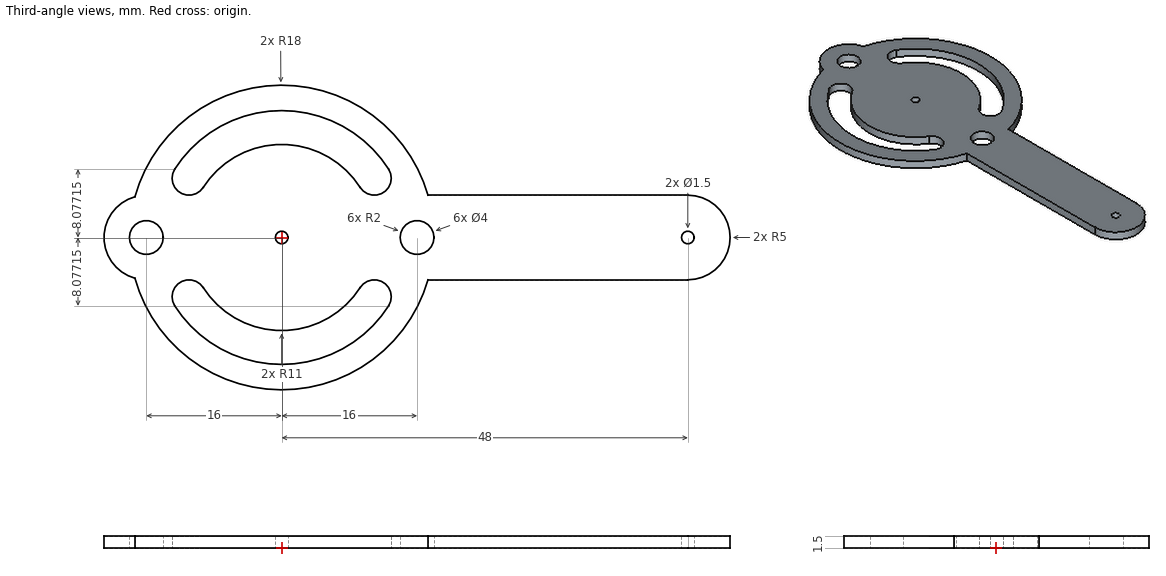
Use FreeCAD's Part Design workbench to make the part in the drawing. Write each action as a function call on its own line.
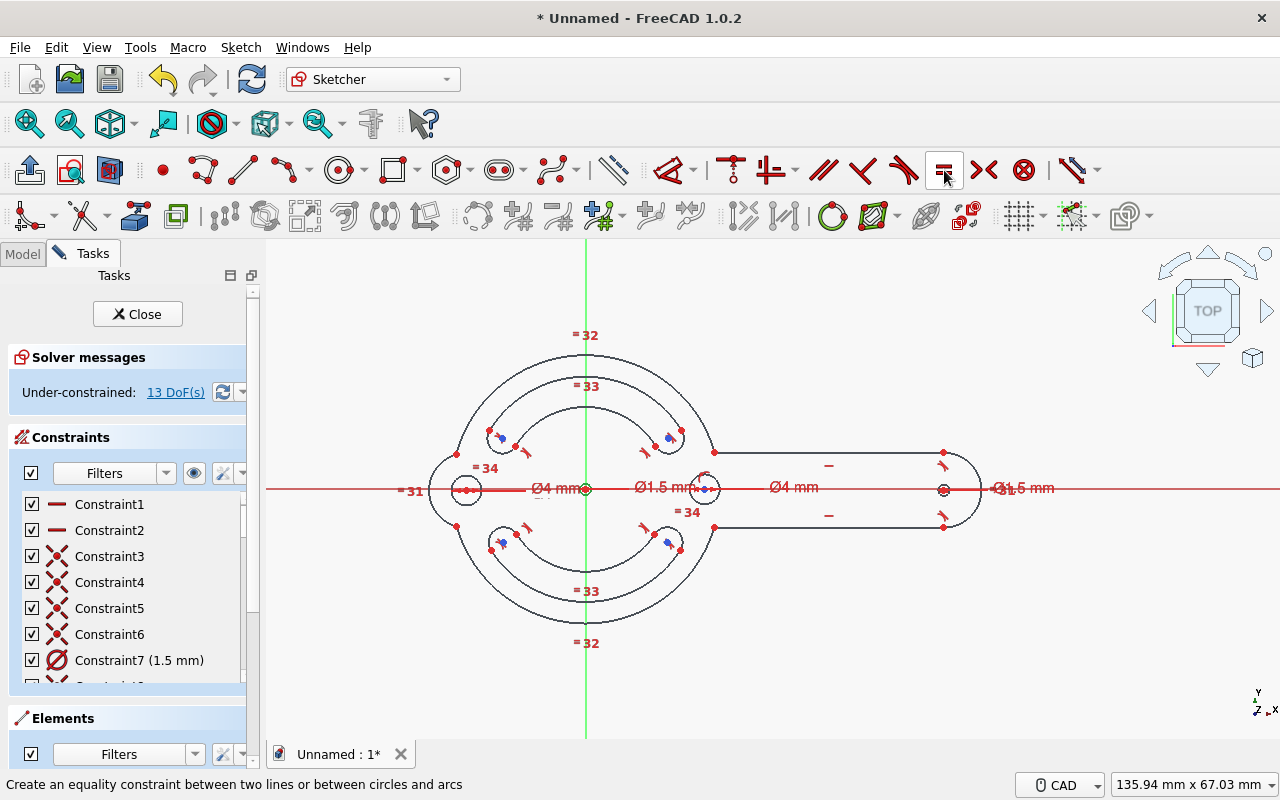
click(944, 490)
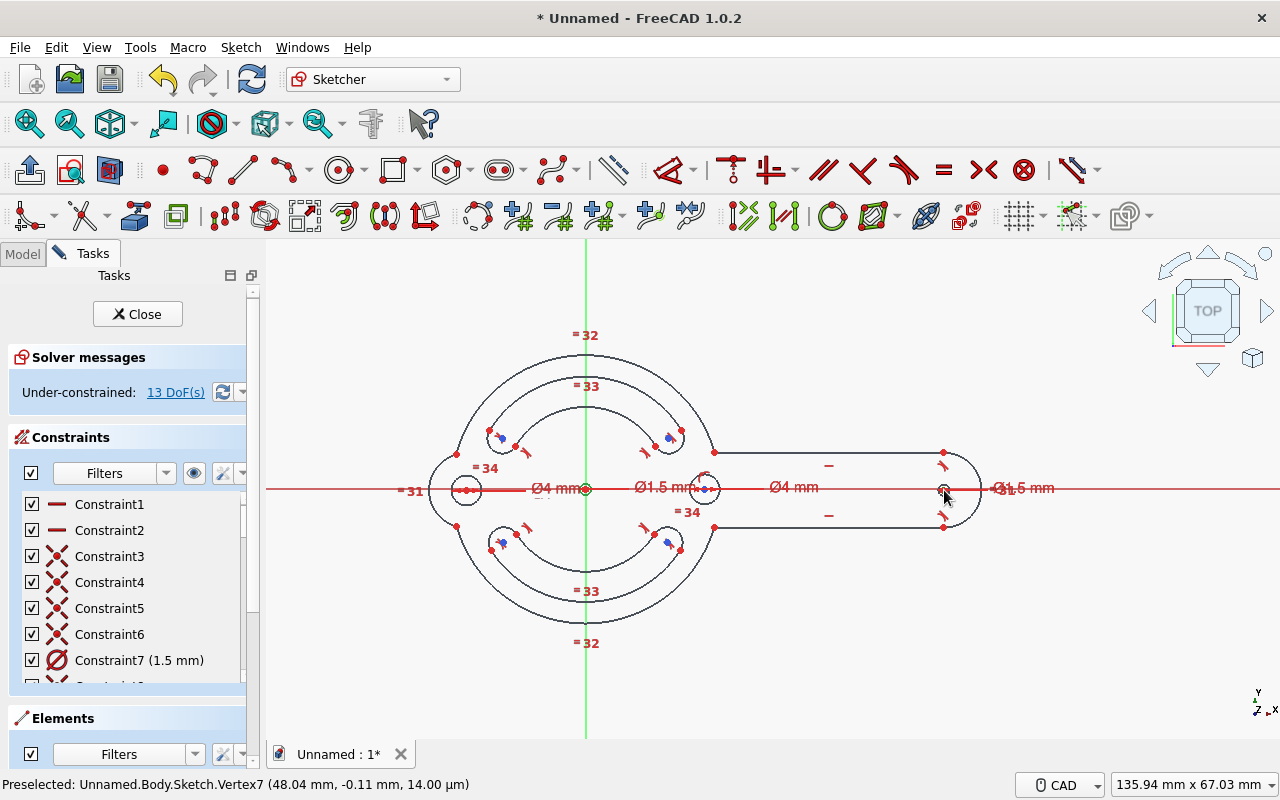
click(353, 489)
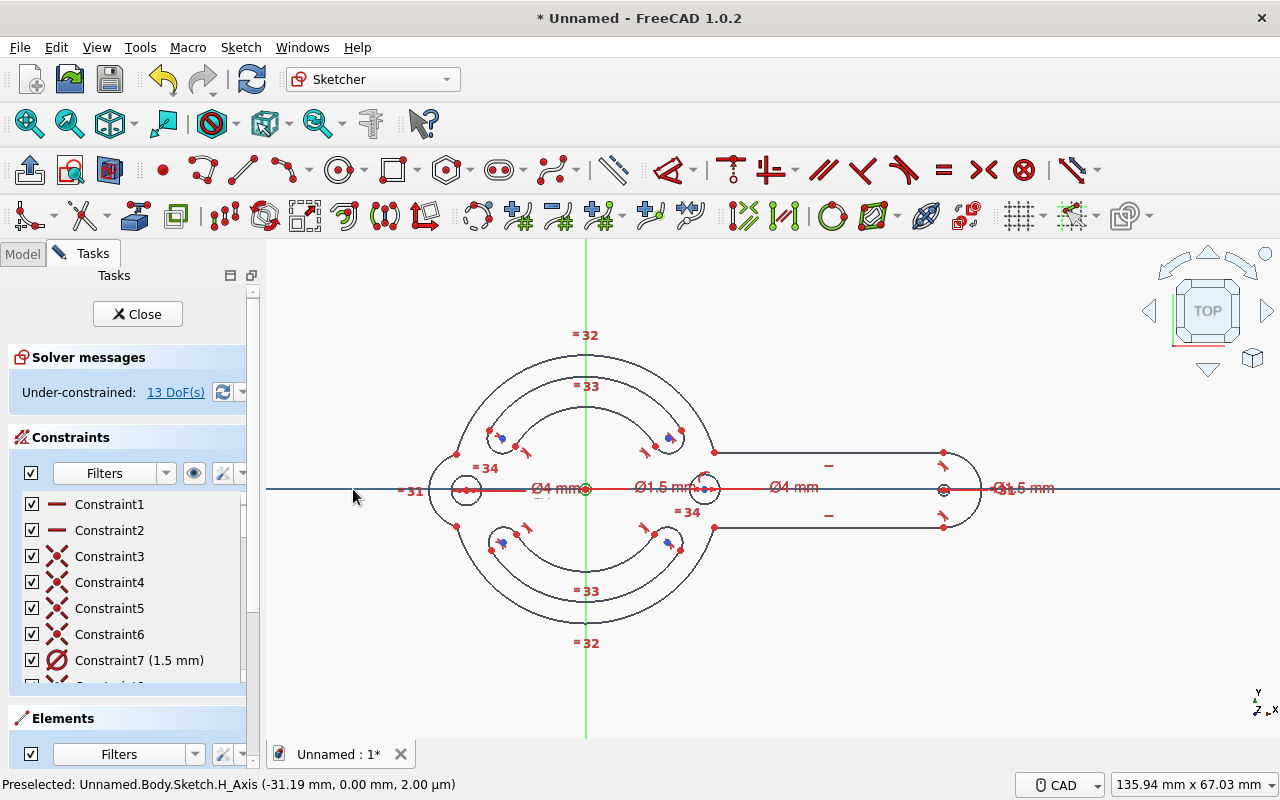
click(732, 170)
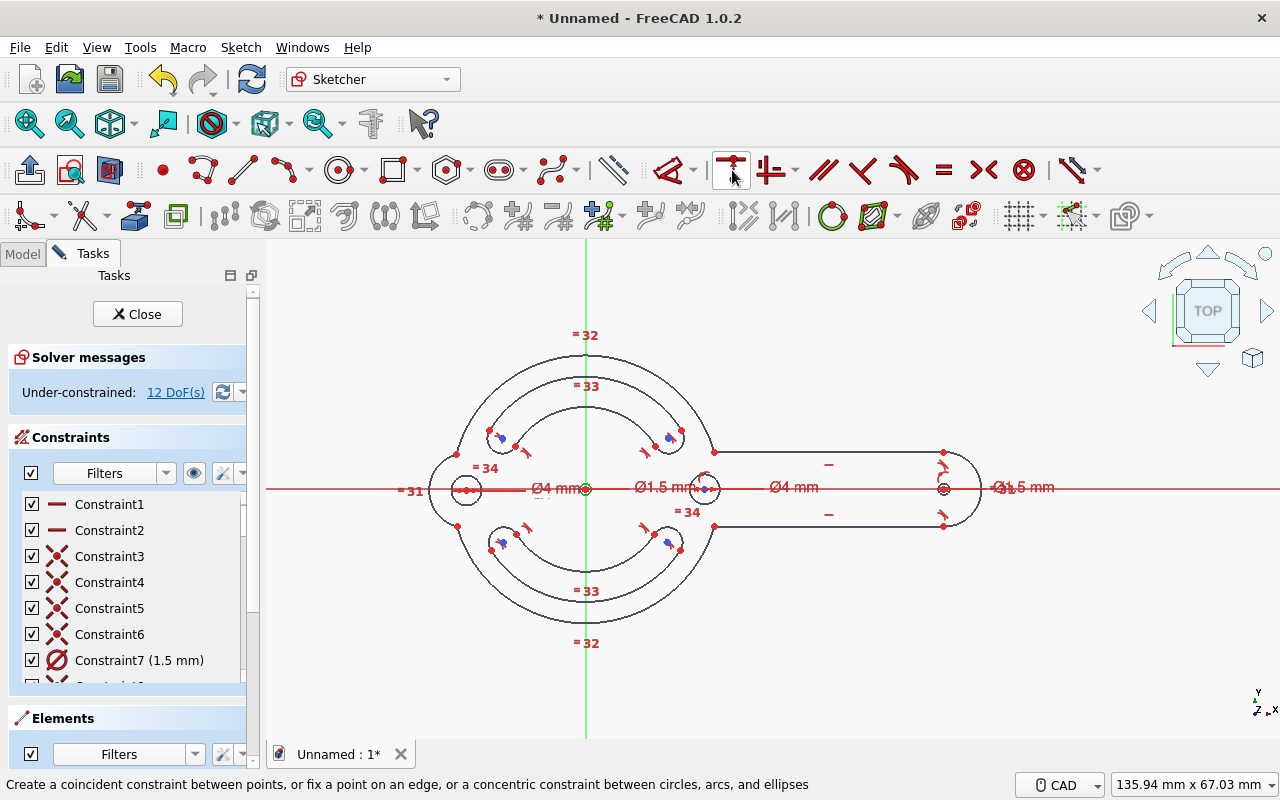
click(467, 491)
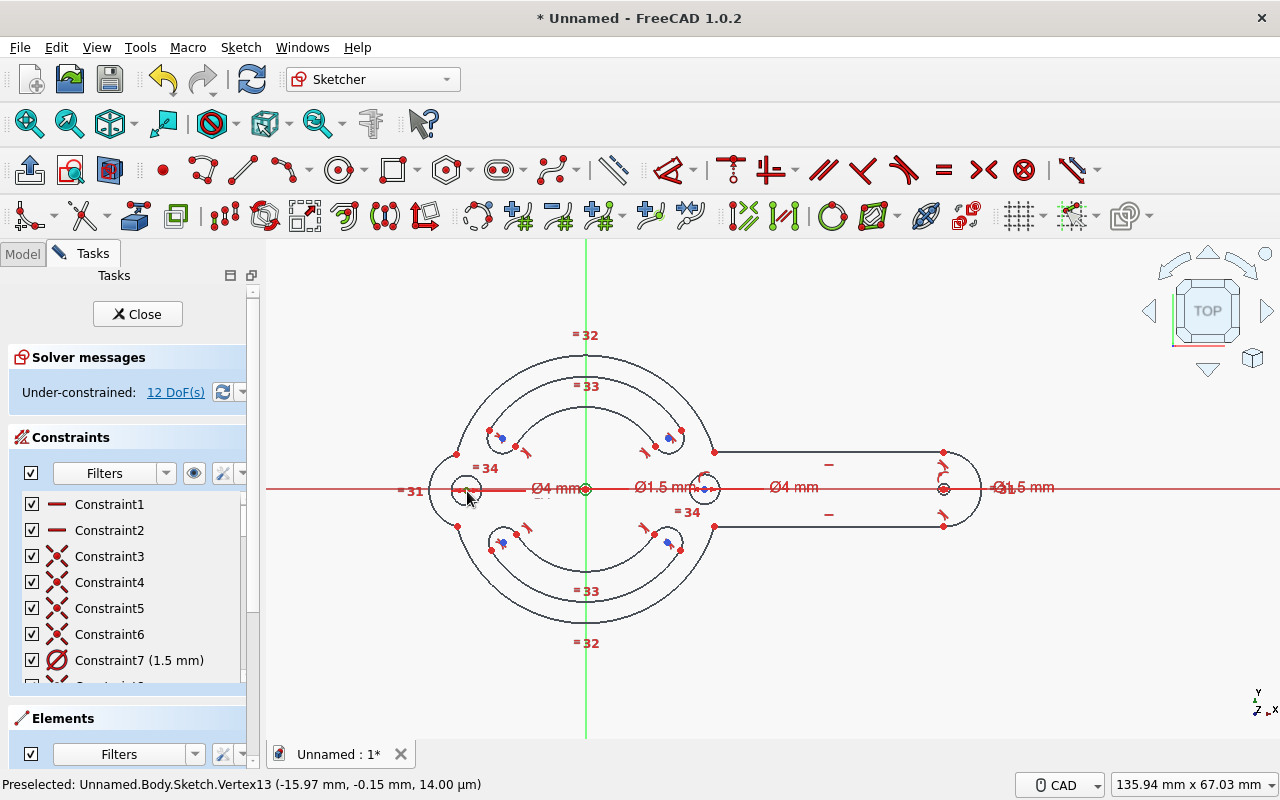
click(353, 489)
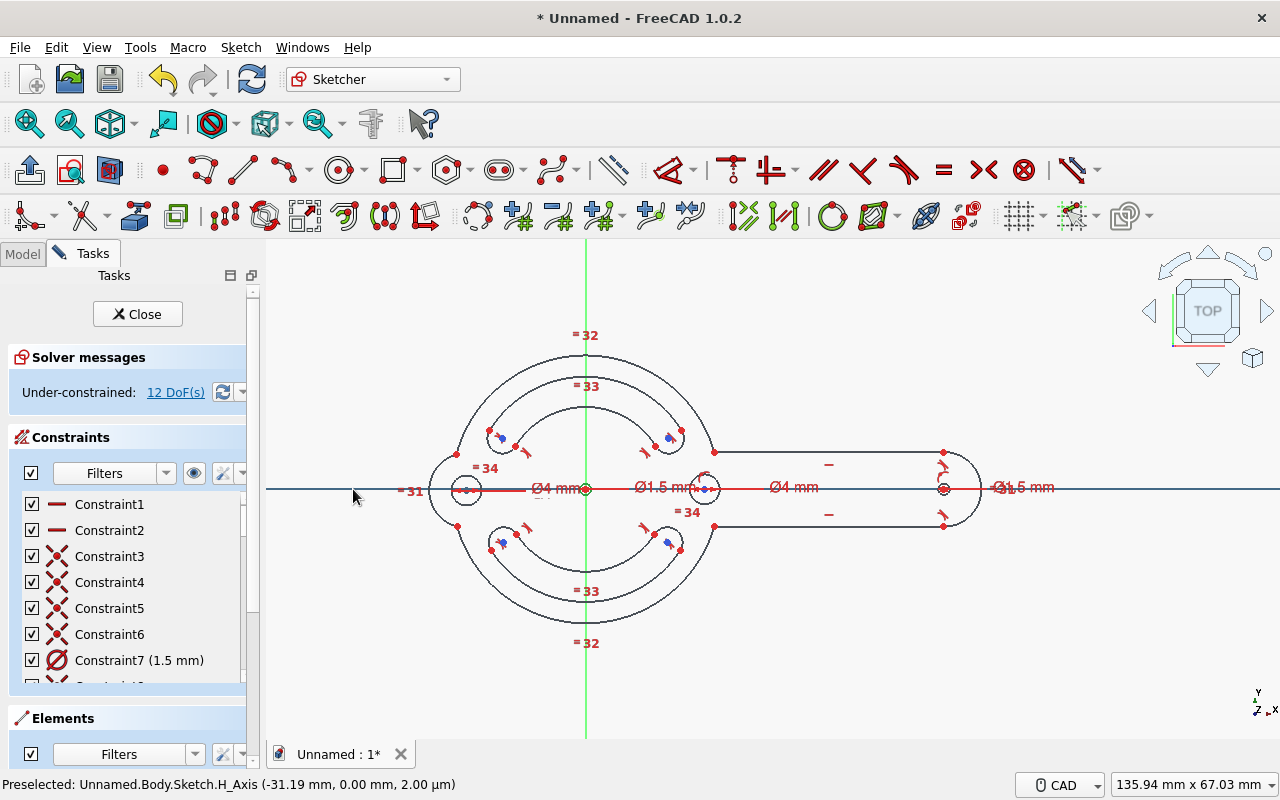
click(732, 170)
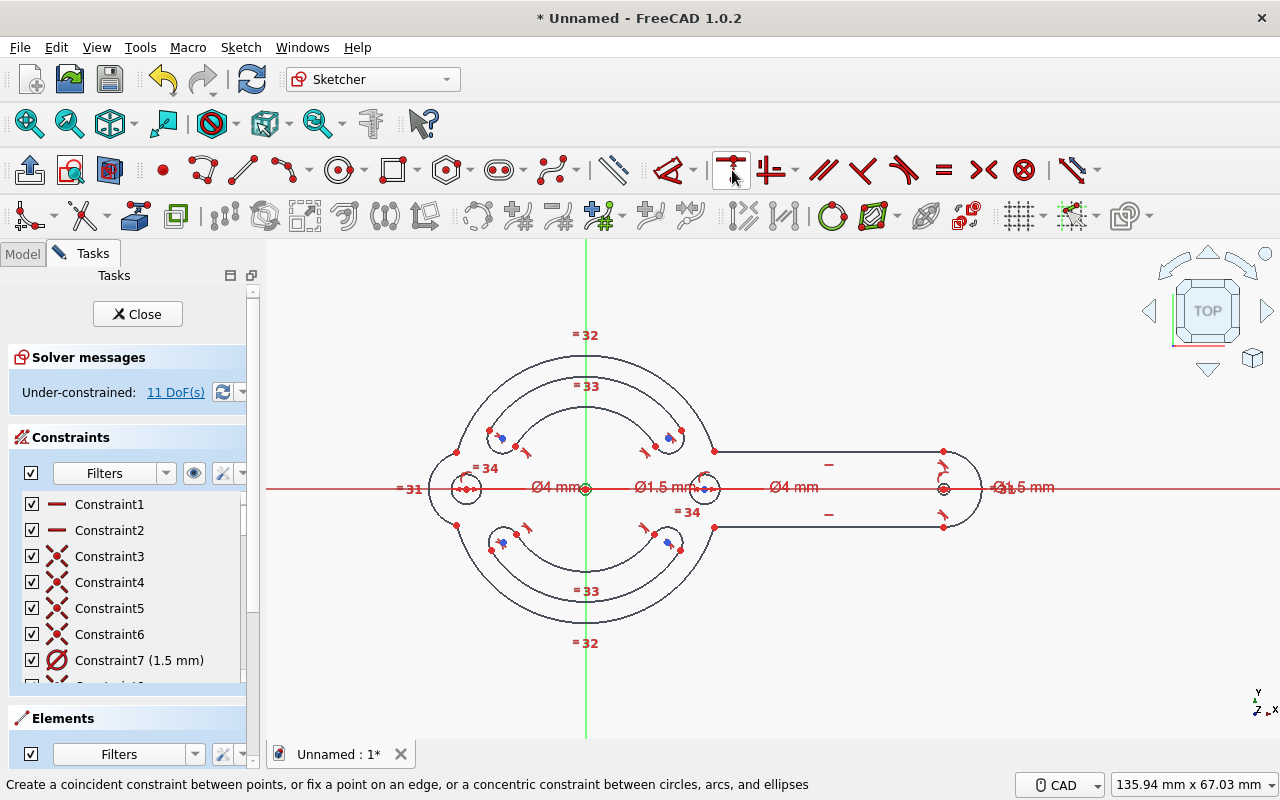
click(668, 170)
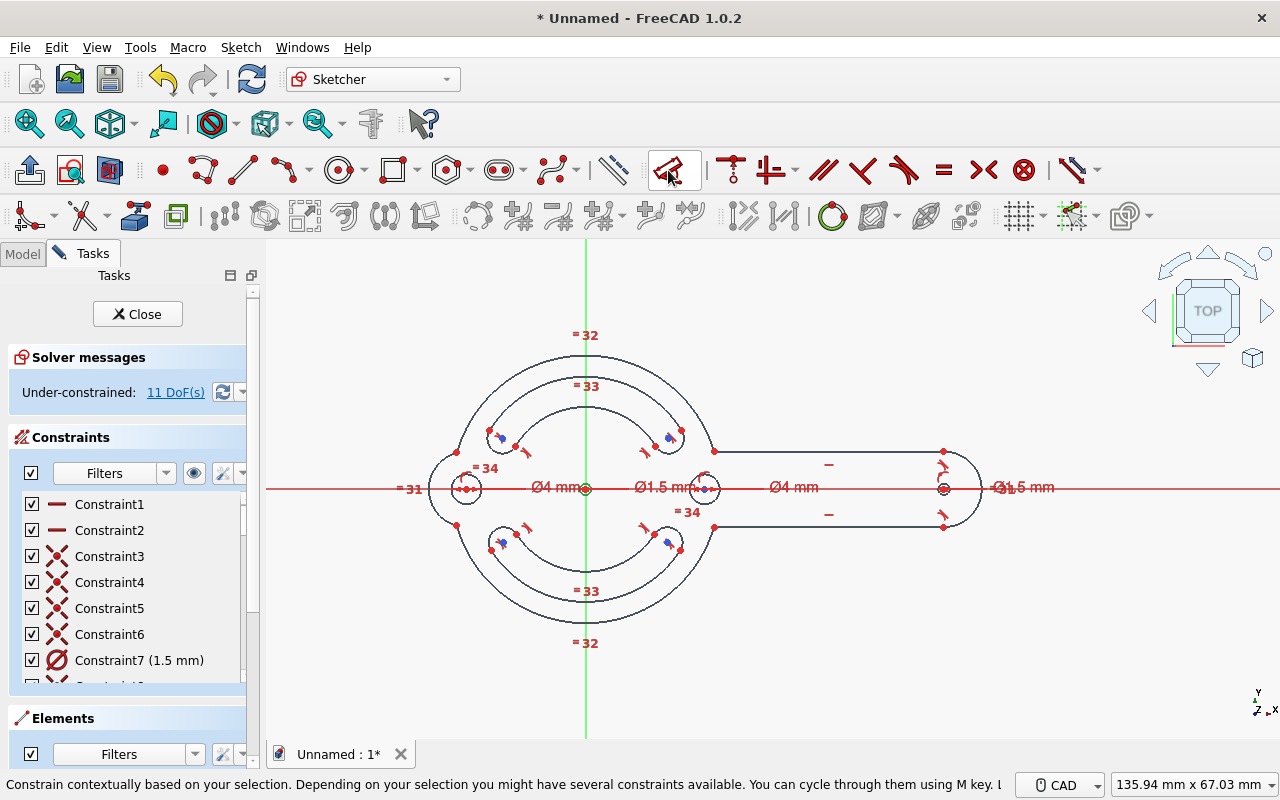
click(974, 512)
click(1000, 531)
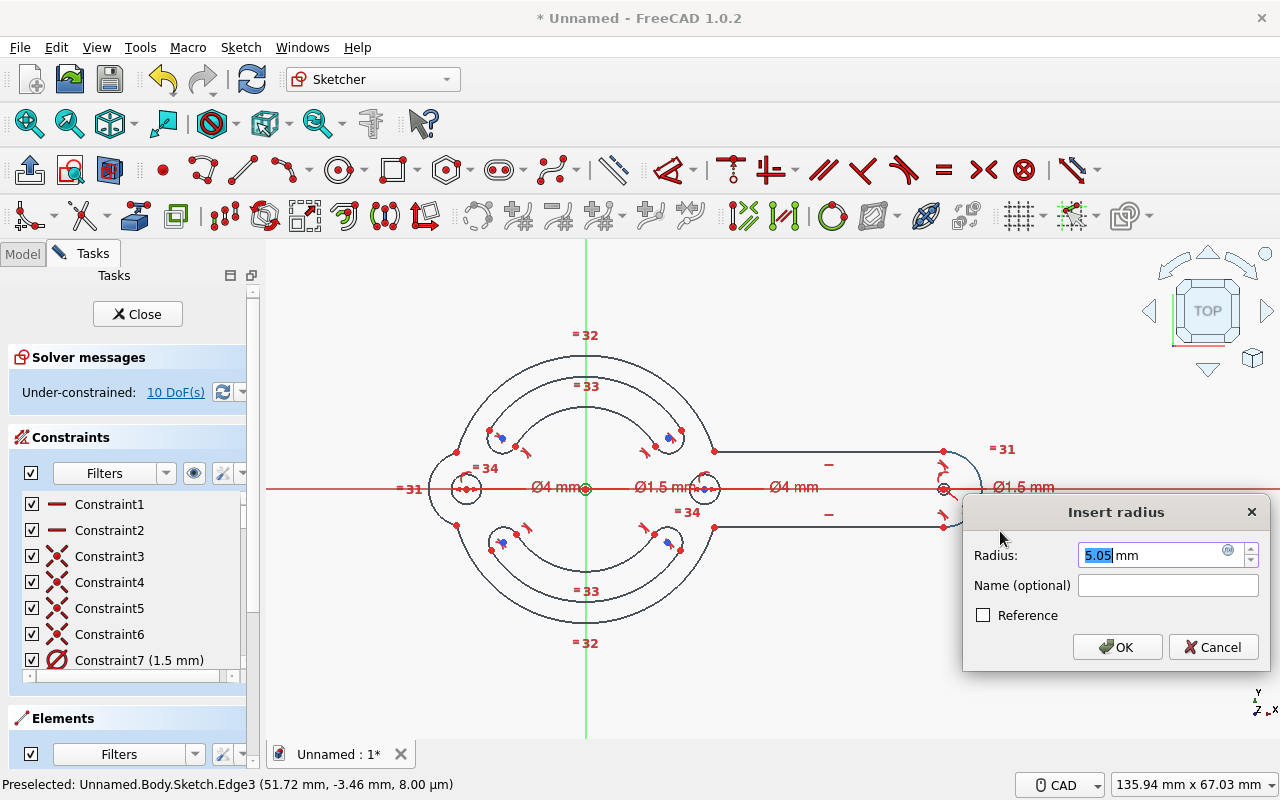
text(5)
key(Return)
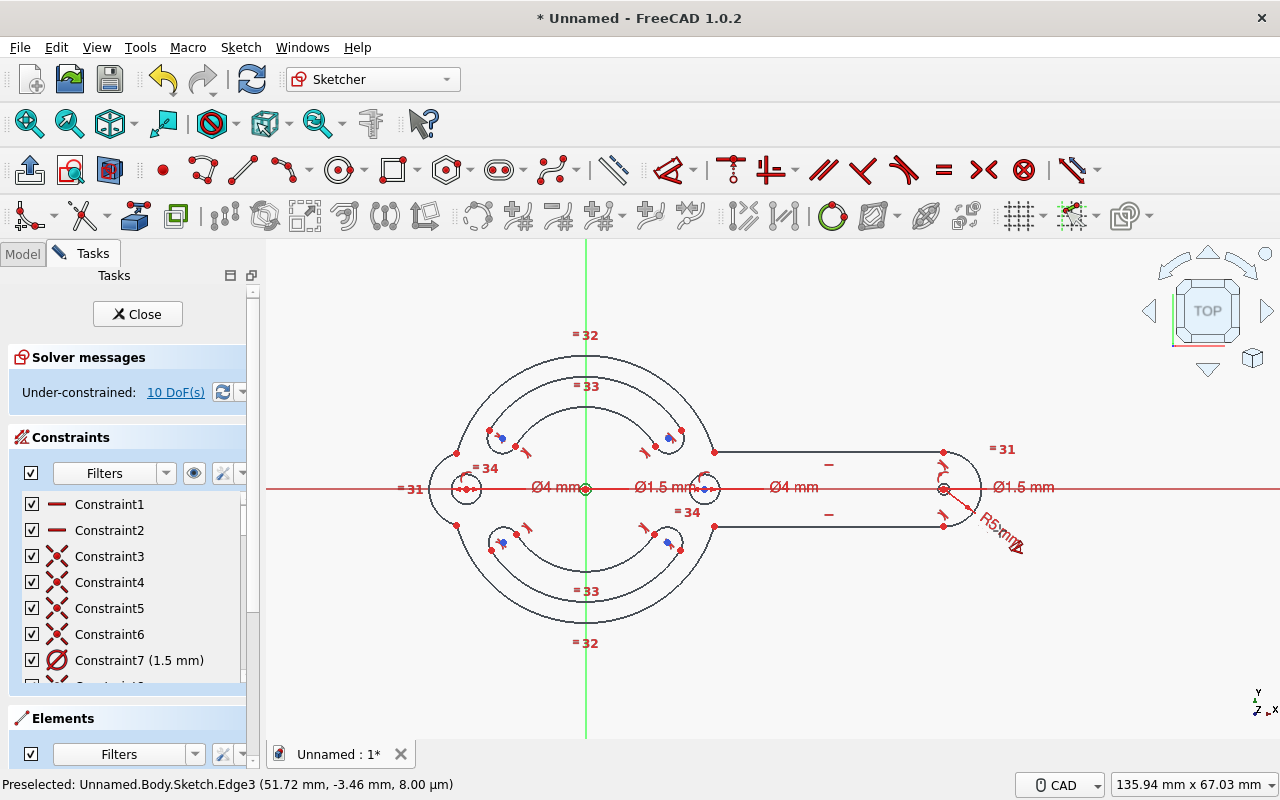
click(651, 373)
click(667, 345)